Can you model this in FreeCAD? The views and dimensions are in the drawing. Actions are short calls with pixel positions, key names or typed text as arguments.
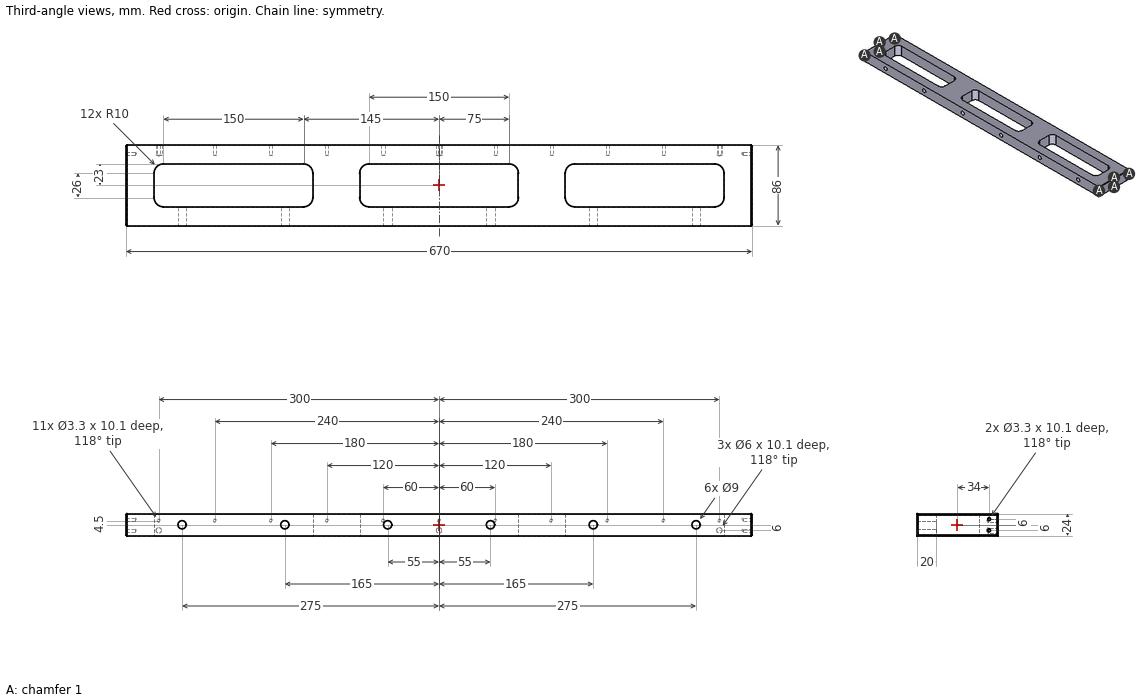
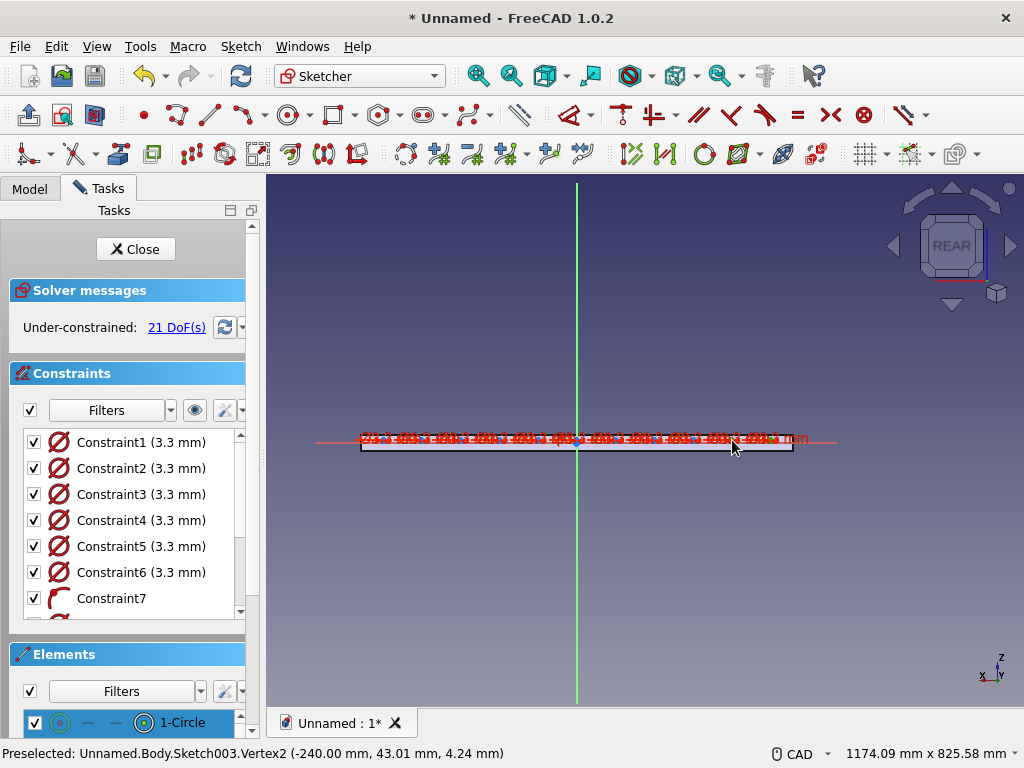
click(676, 116)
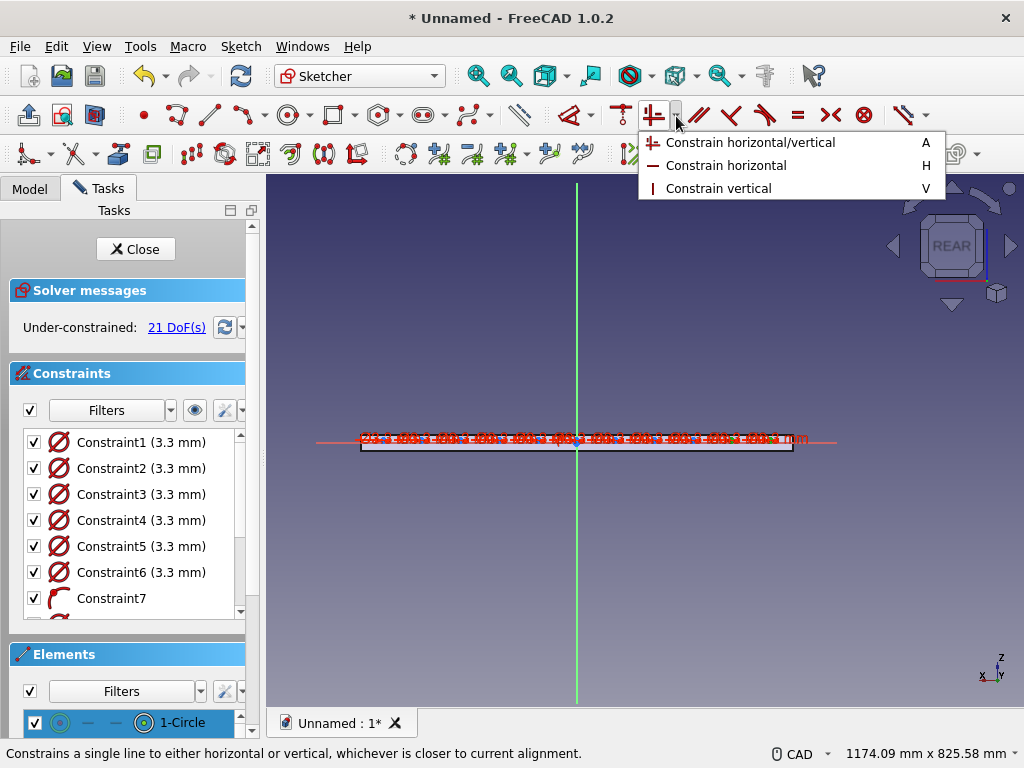
click(792, 166)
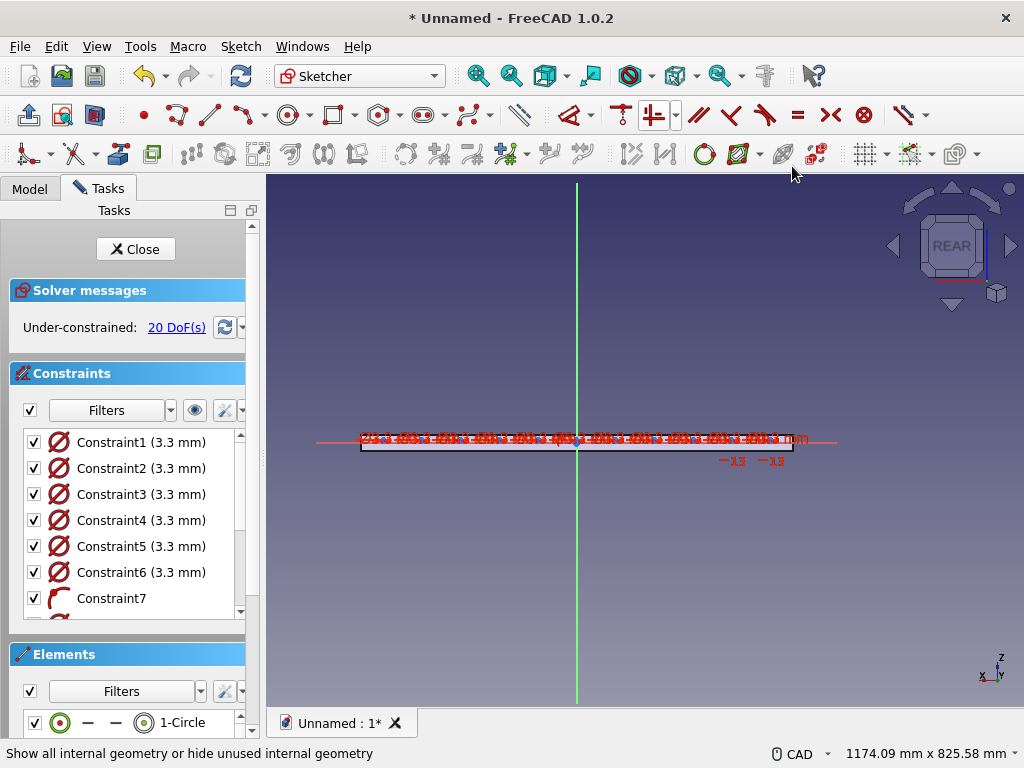
click(732, 440)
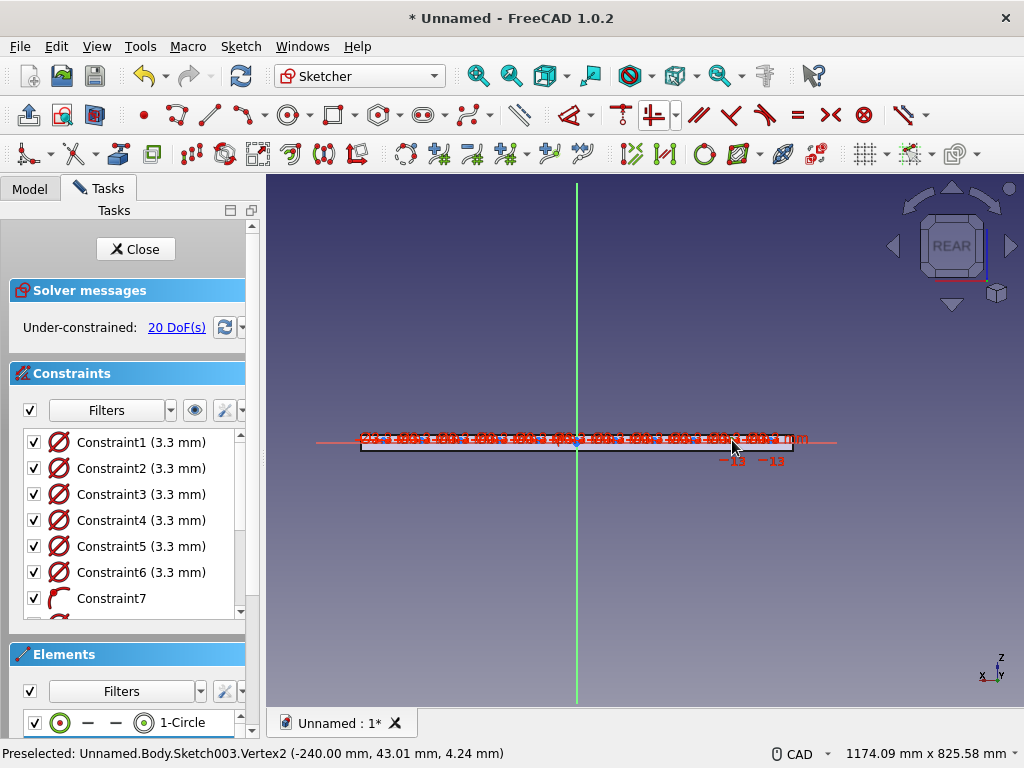
click(693, 440)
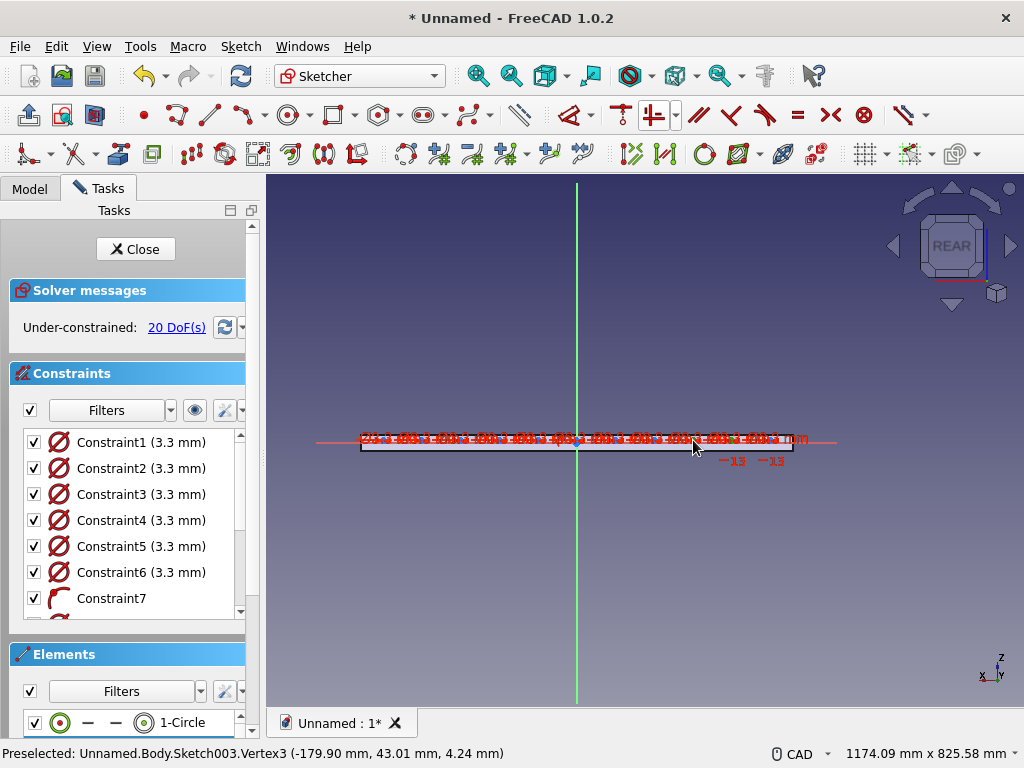
click(676, 116)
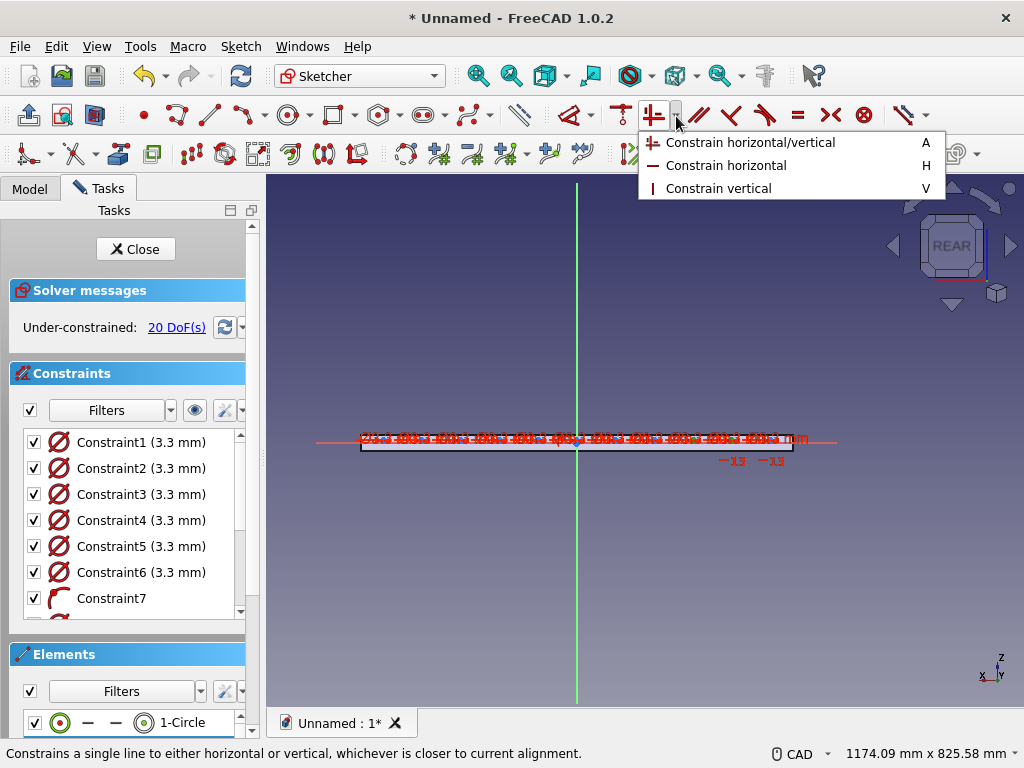
click(792, 166)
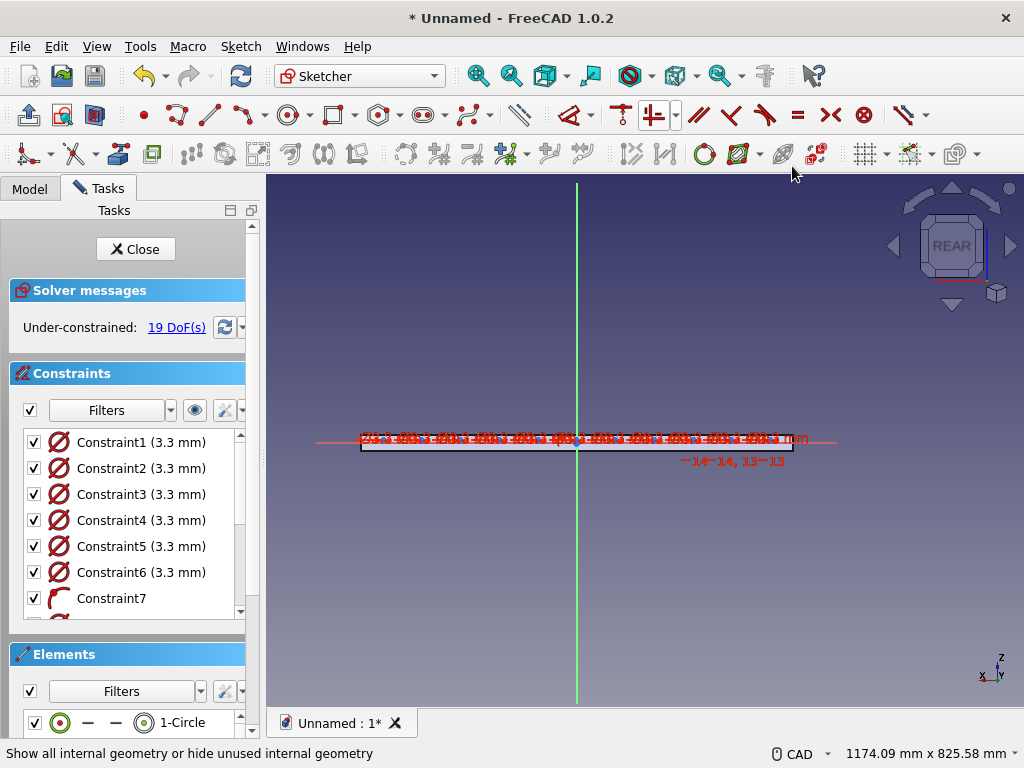
click(693, 440)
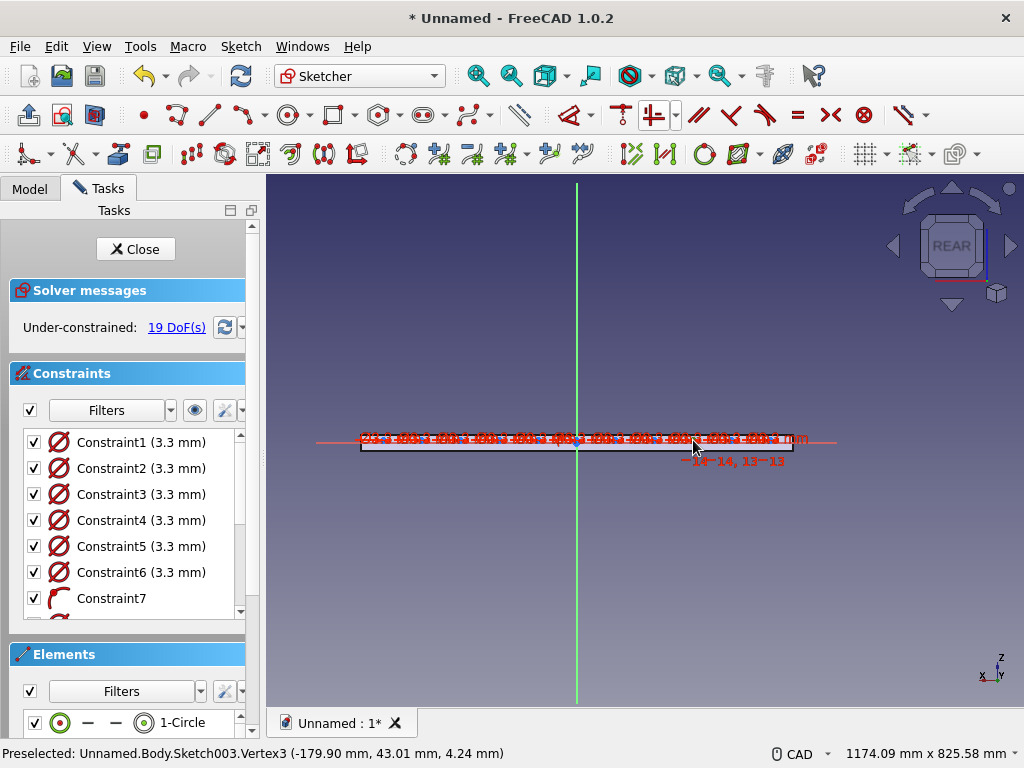
click(654, 440)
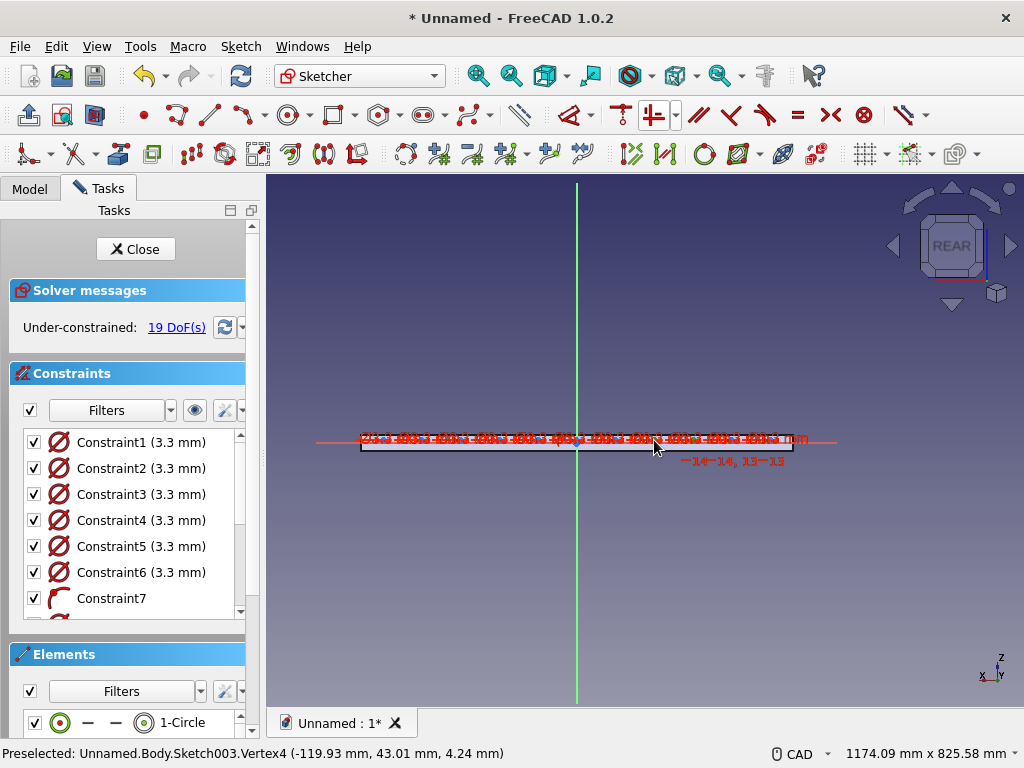
key(h)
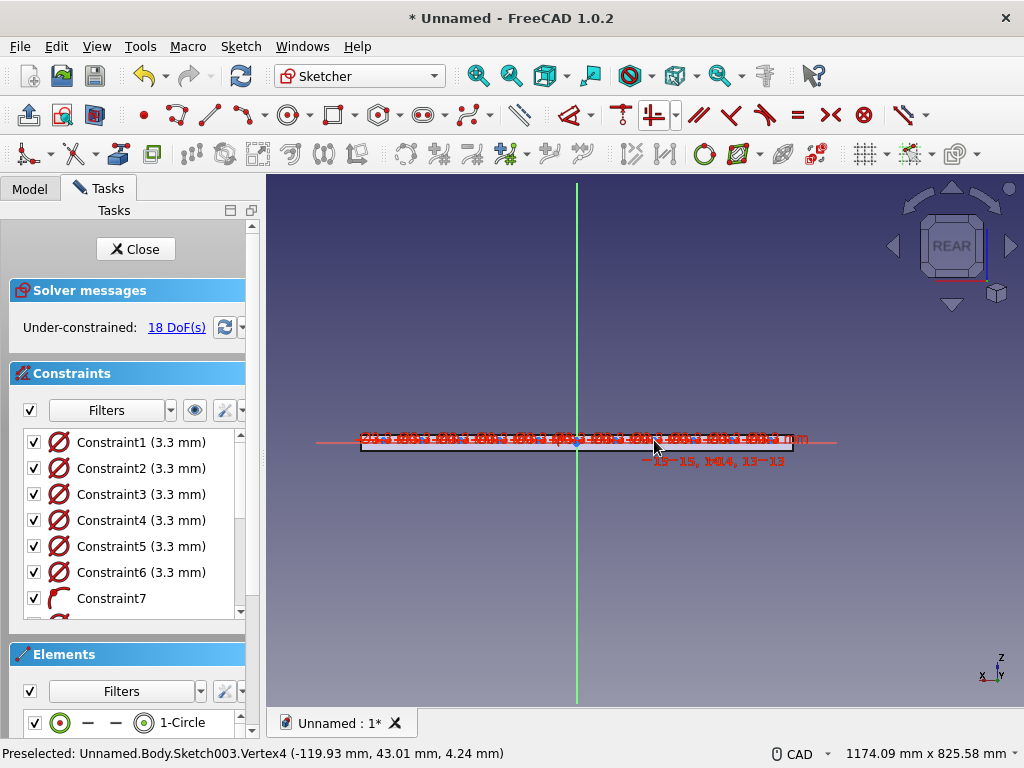
click(654, 440)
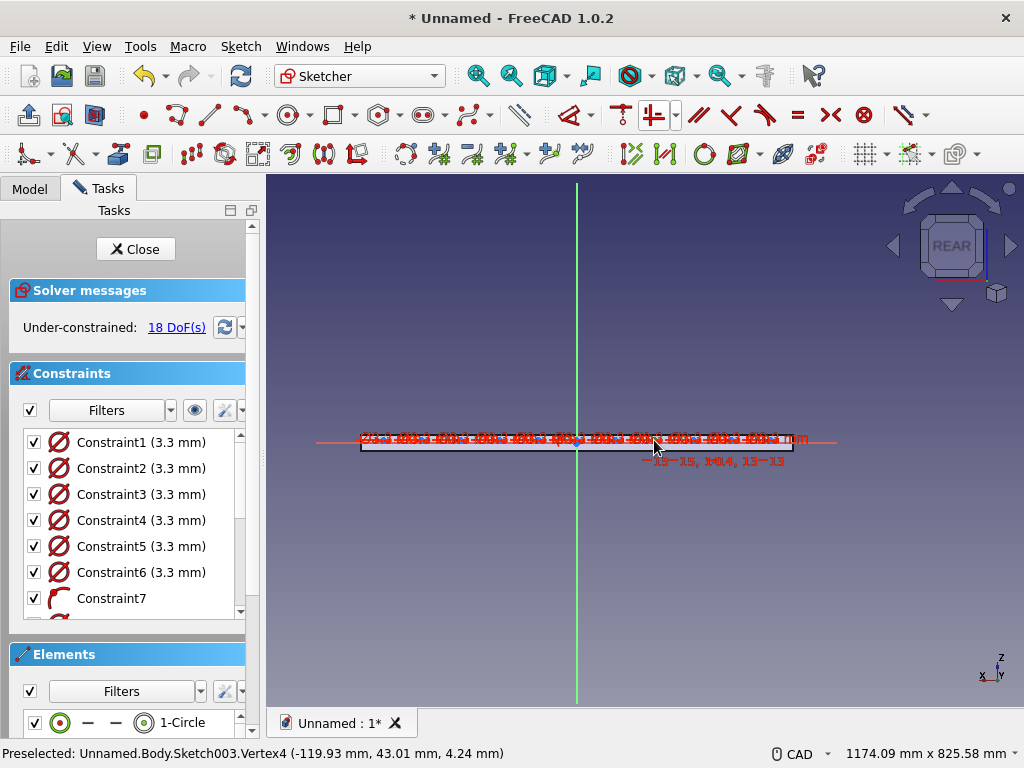
click(616, 440)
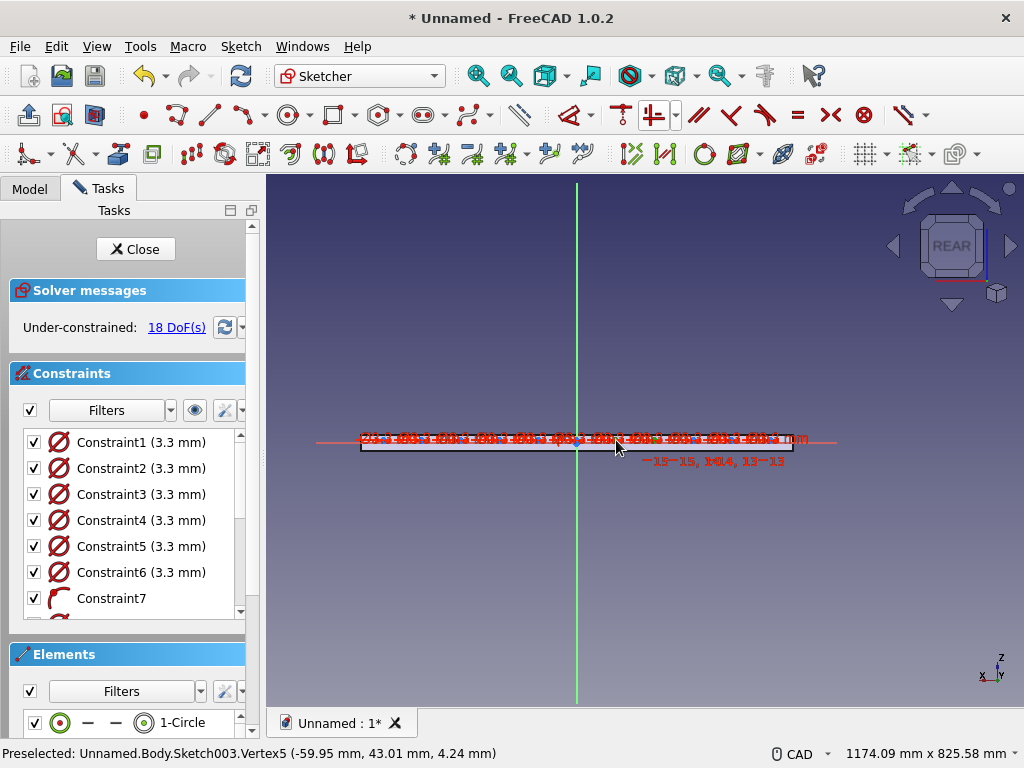
key(h)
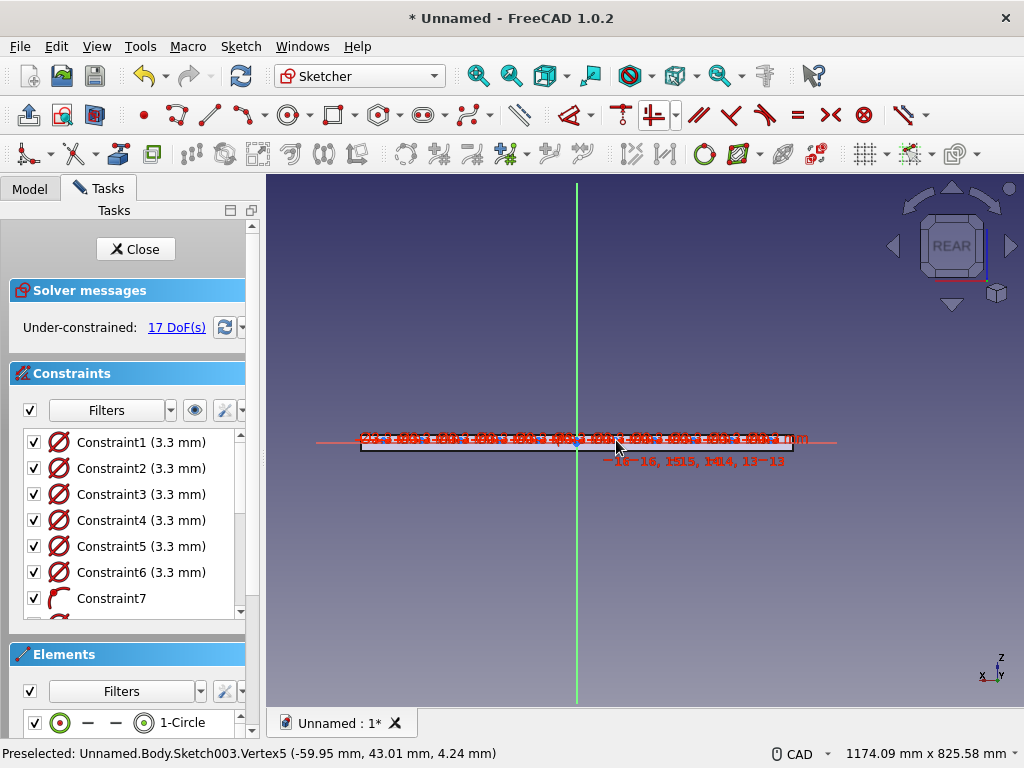
click(616, 440)